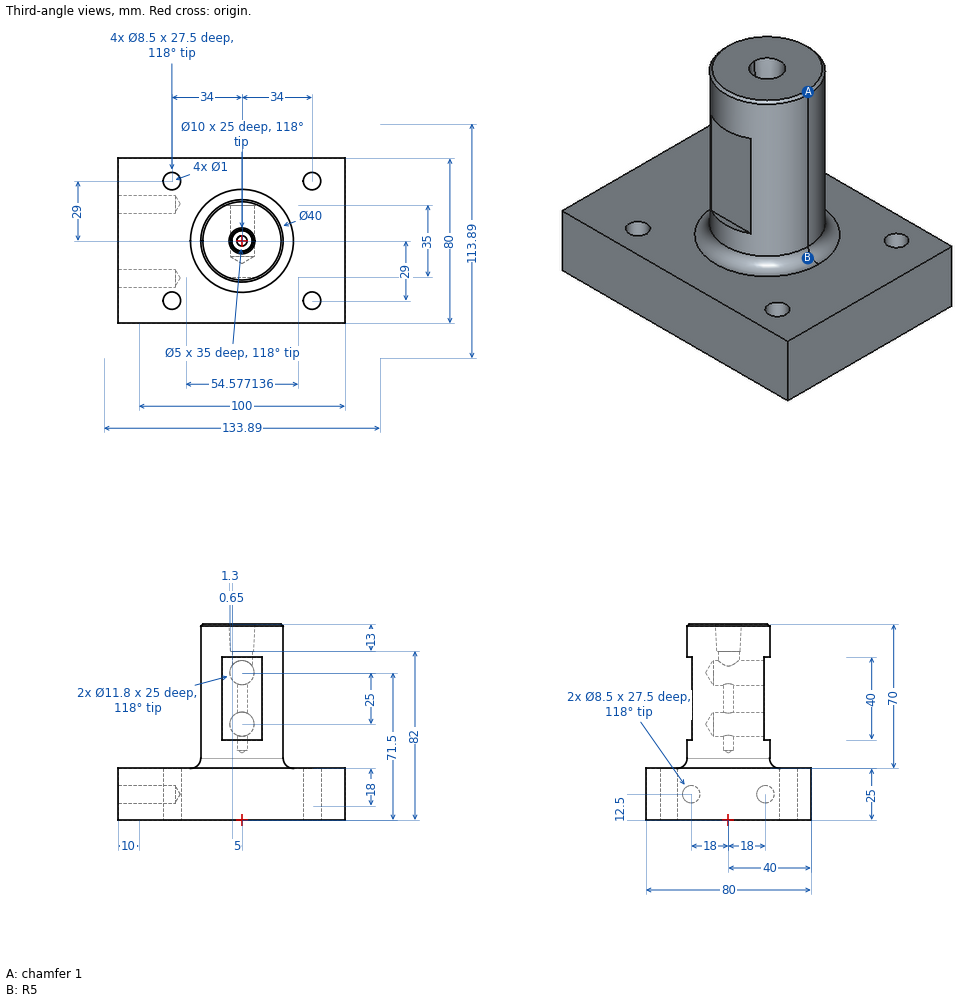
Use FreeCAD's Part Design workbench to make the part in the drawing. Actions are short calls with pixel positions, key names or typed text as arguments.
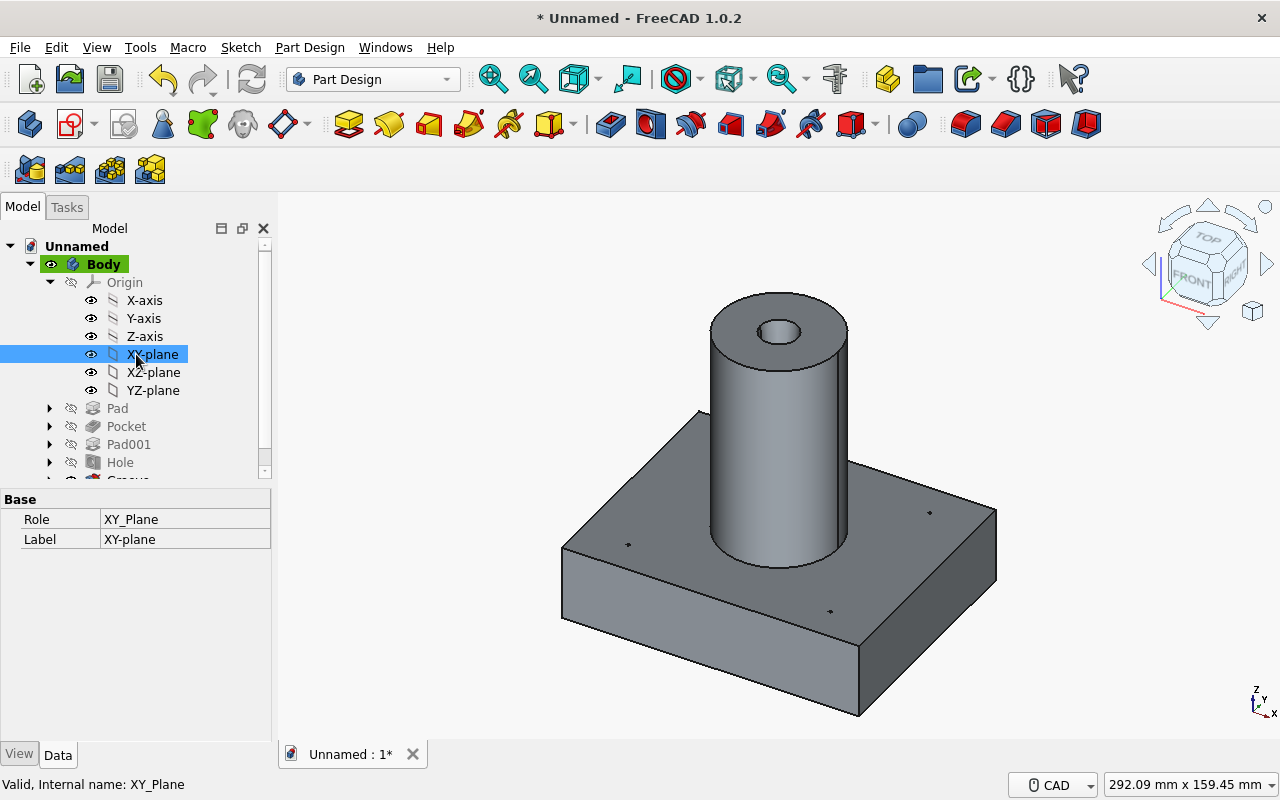
click(284, 124)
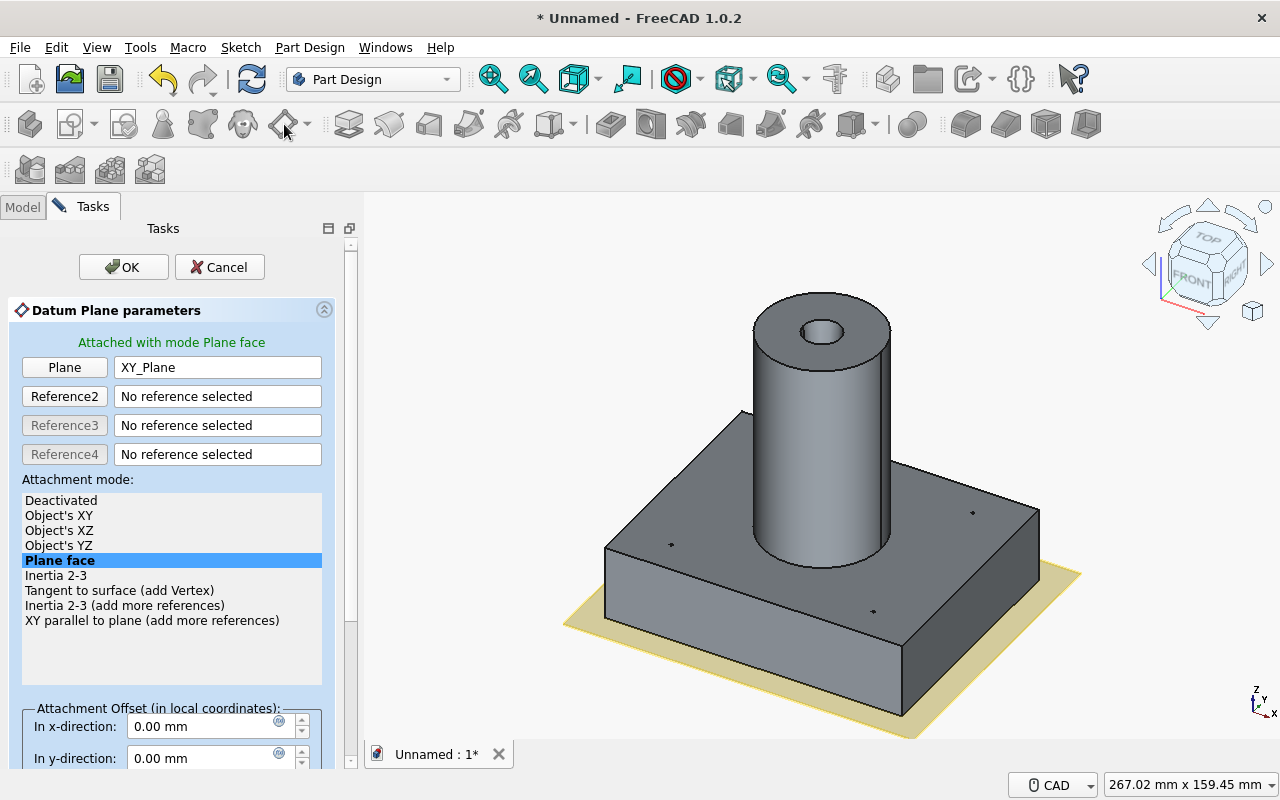
scroll(351, 503, down, 2)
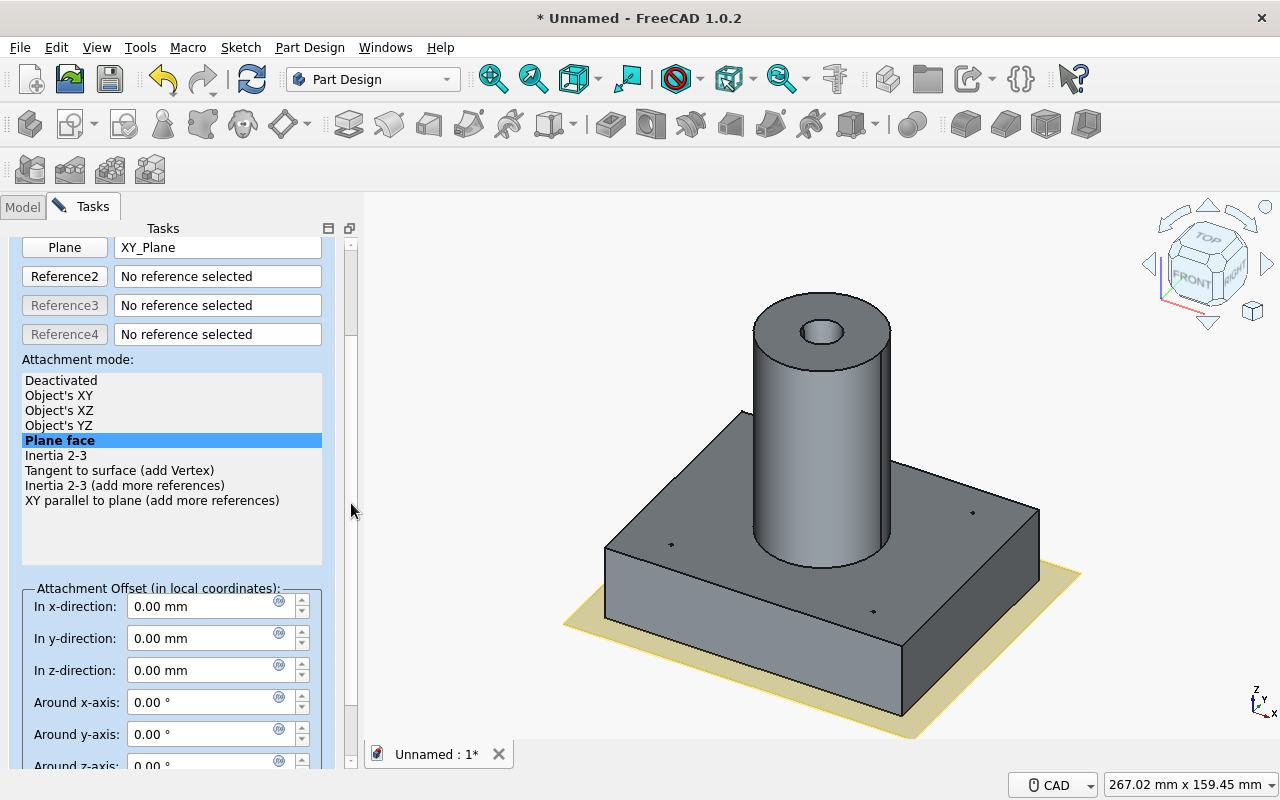
triple_click(210, 670)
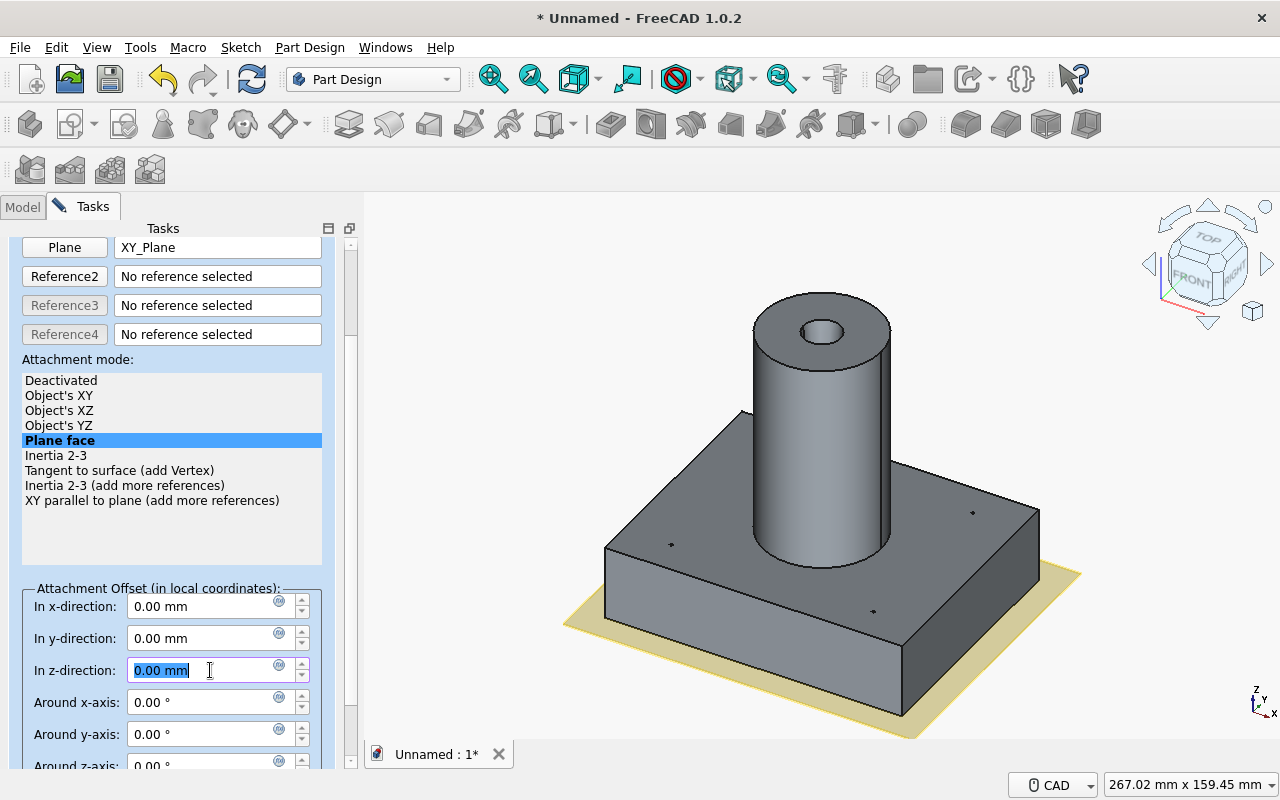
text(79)
key(Tab)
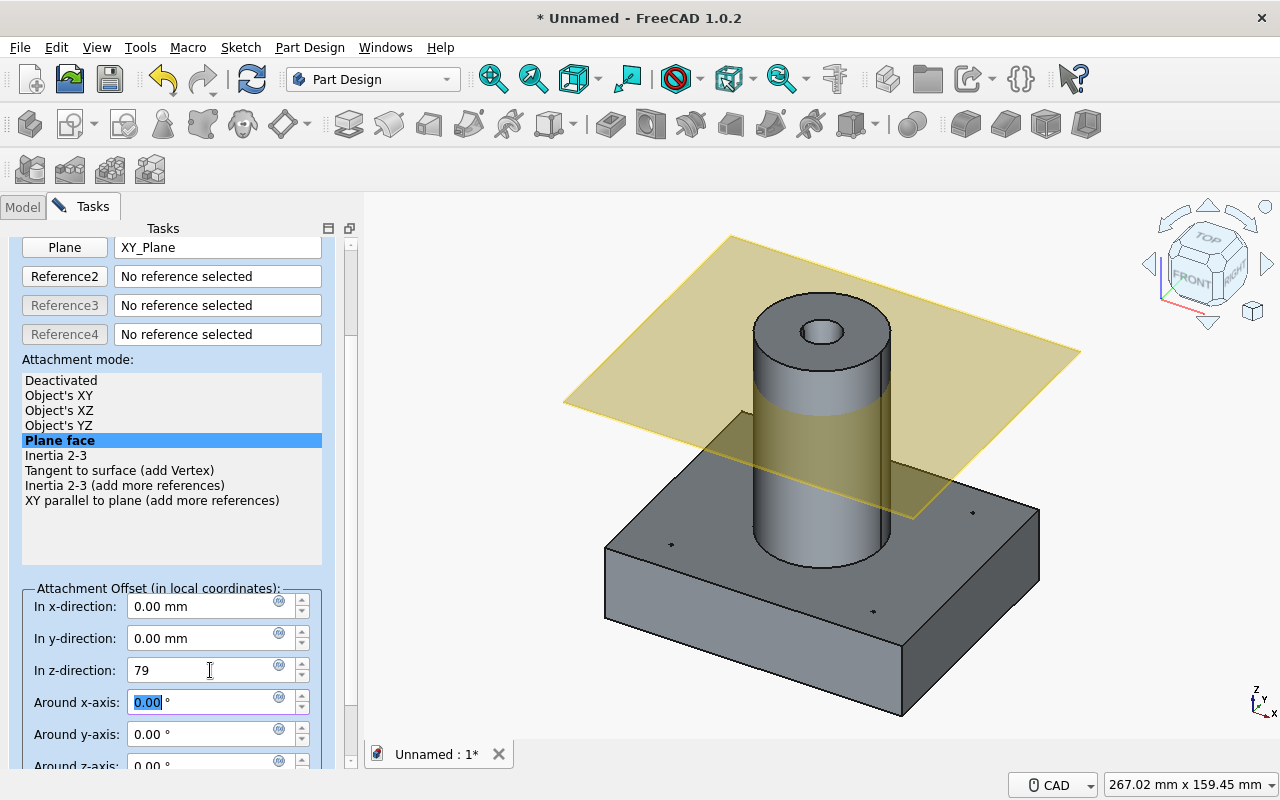
scroll(351, 503, up, 3)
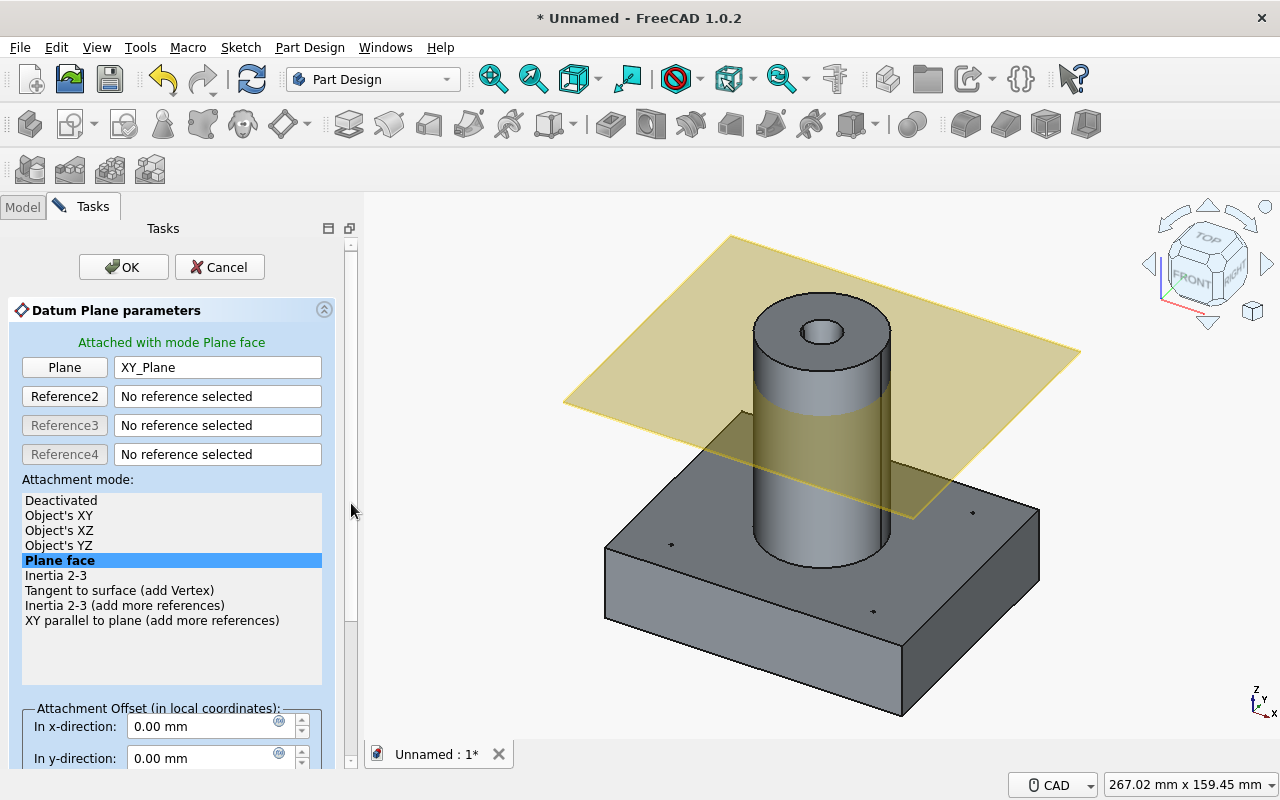
click(124, 267)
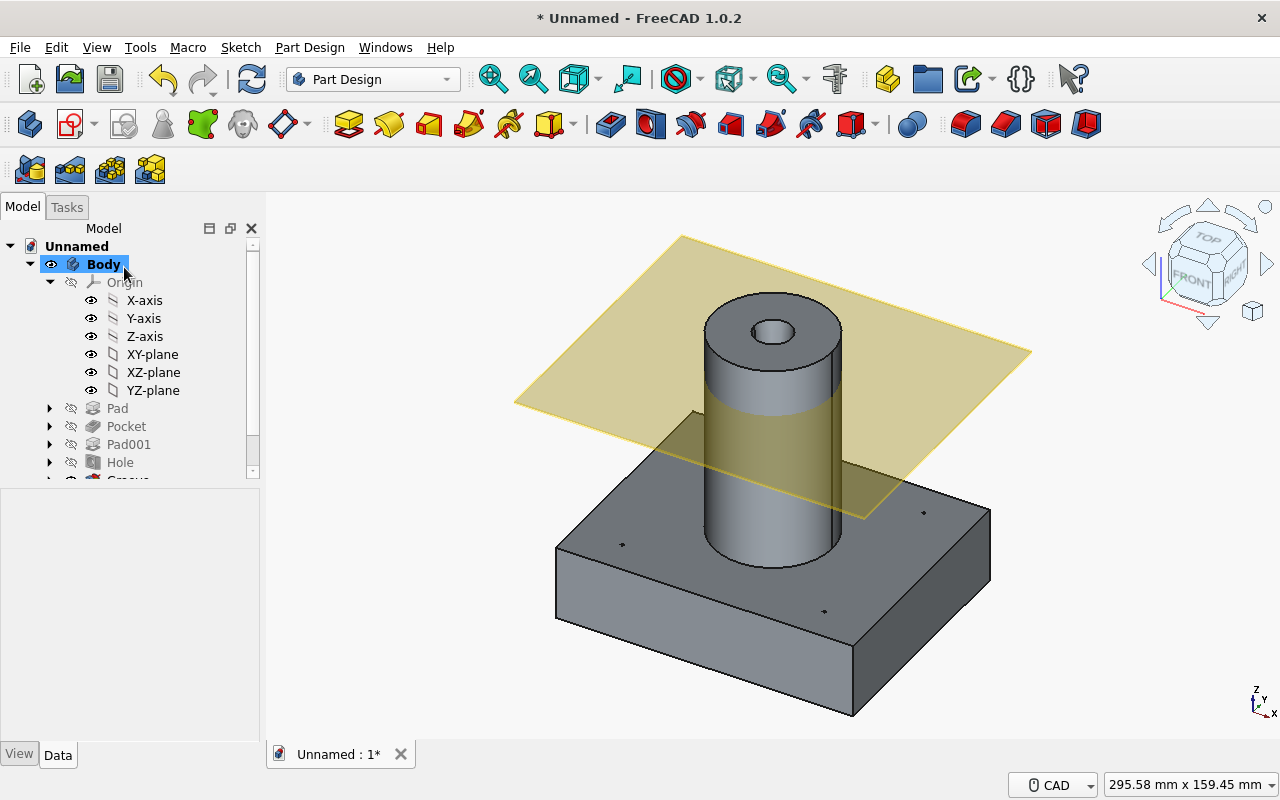
scroll(100, 350, down, 3)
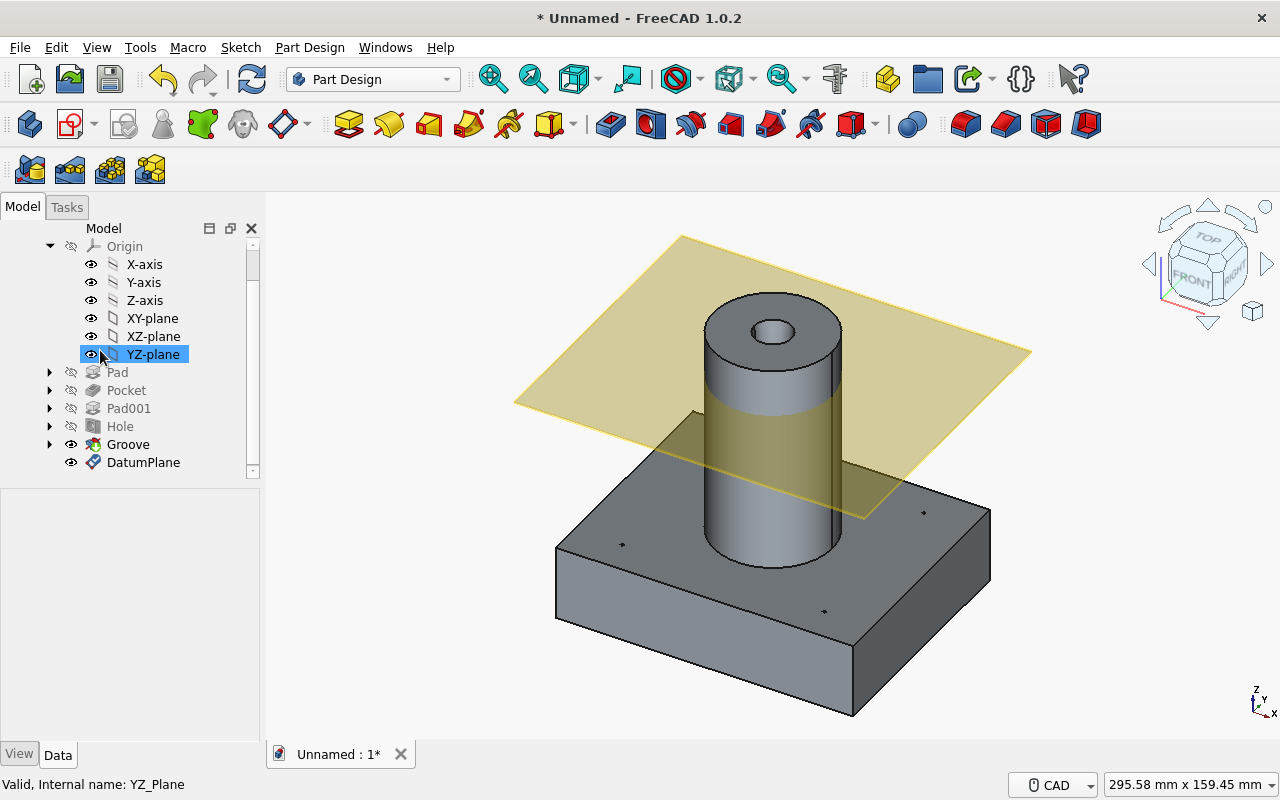
click(116, 462)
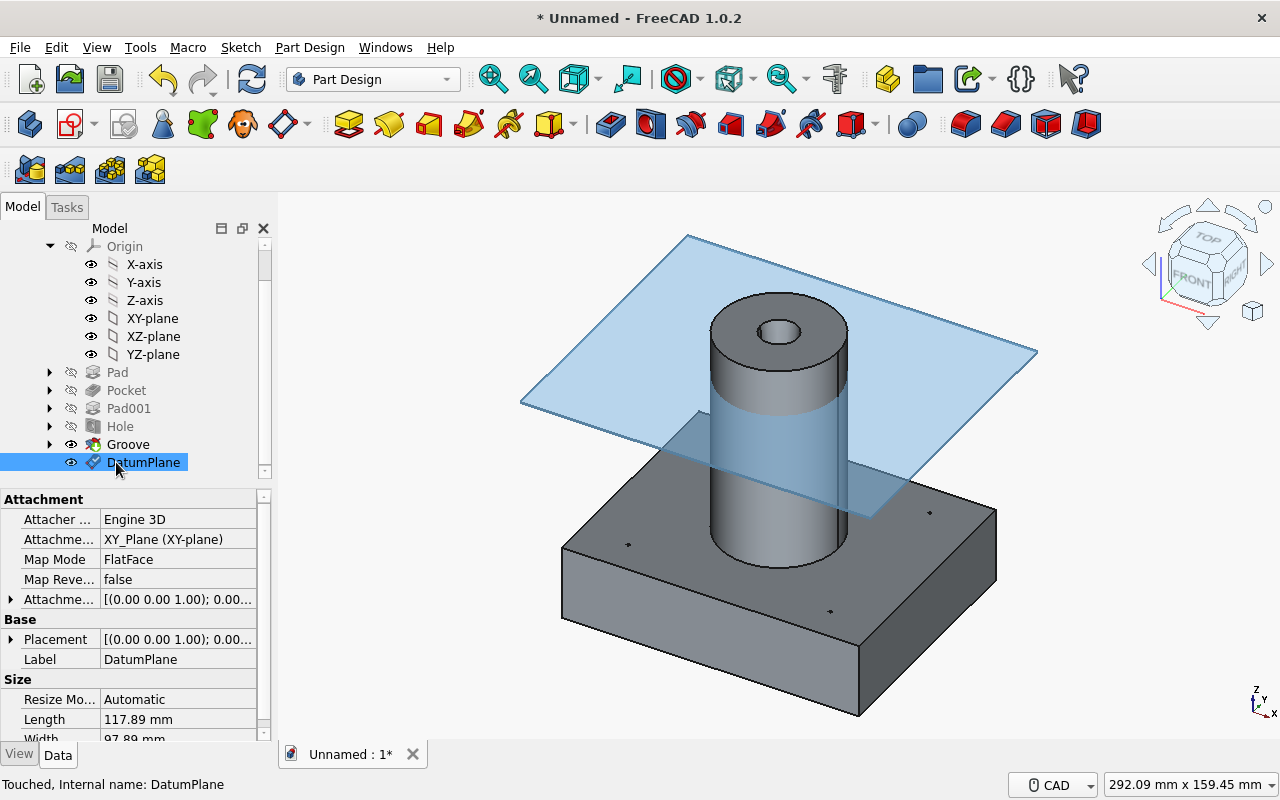
click(70, 124)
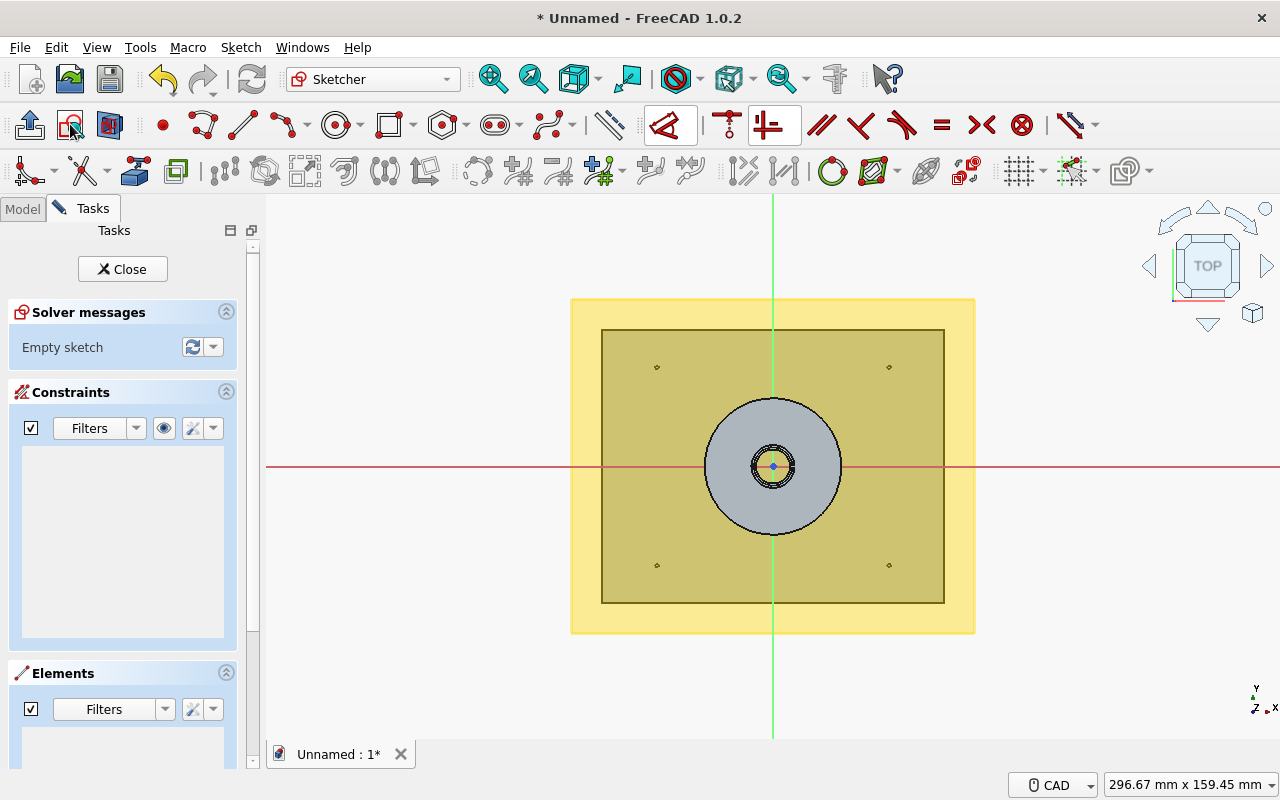
click(110, 126)